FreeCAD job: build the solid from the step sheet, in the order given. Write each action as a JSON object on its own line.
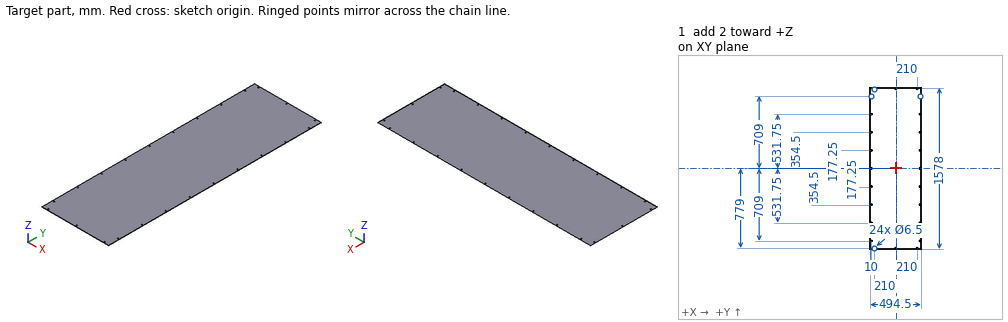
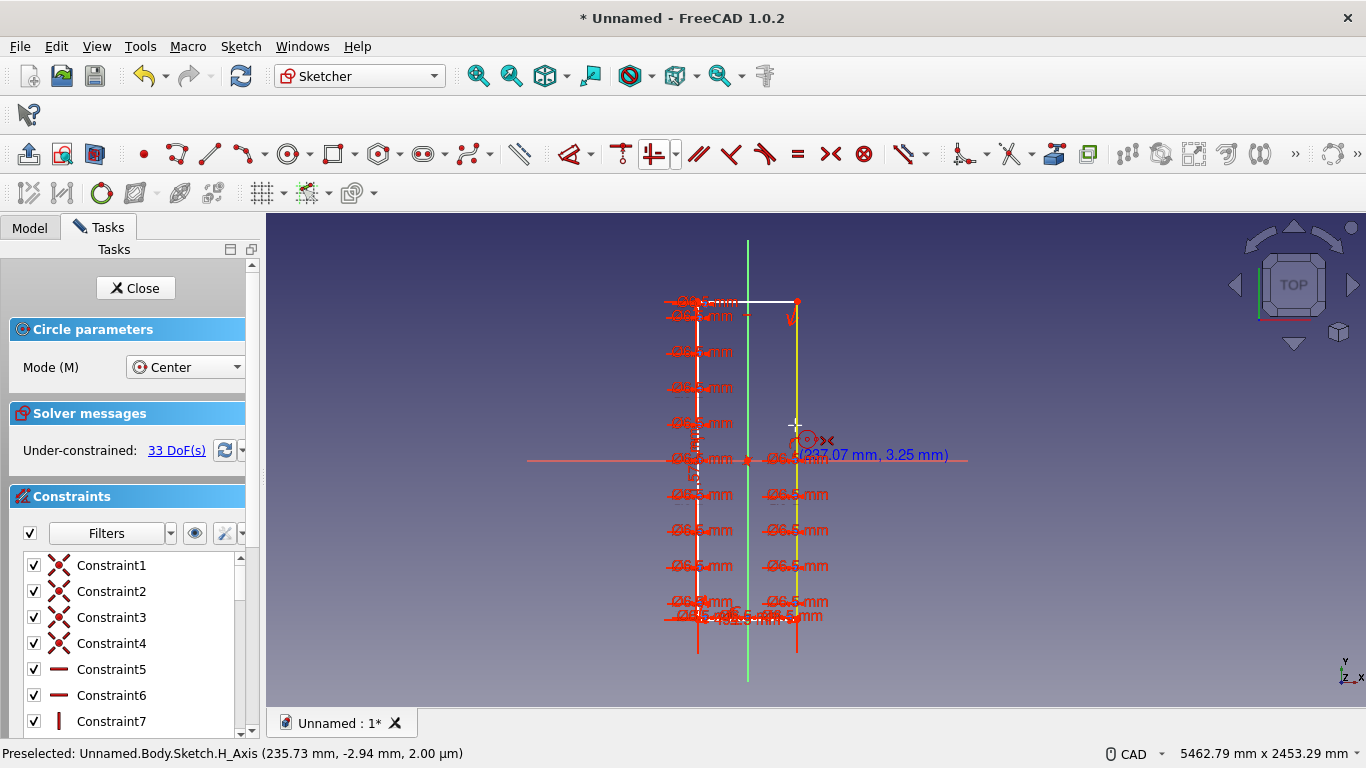
{"action": "scroll", "coordinate": [795, 425], "scroll_direction": "up", "scroll_amount": 11}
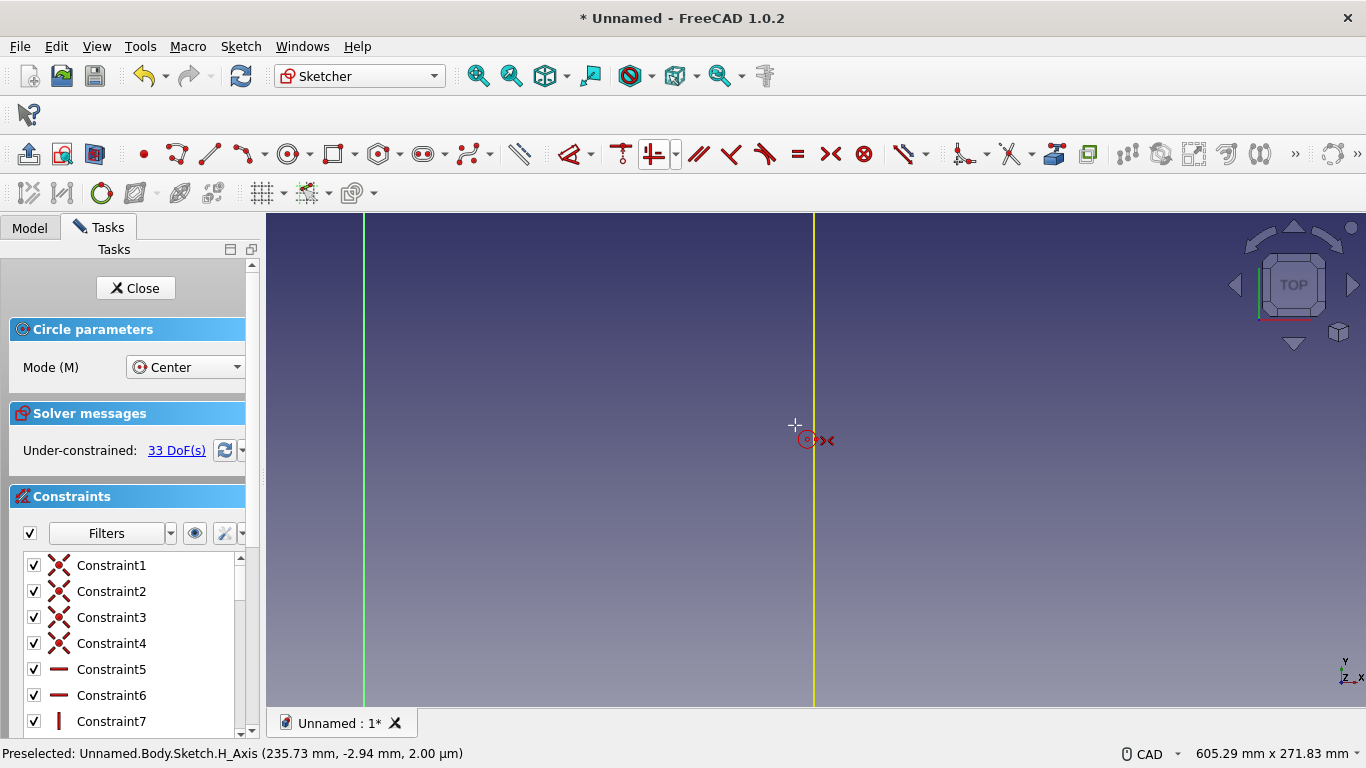
{"action": "left_click", "coordinate": [795, 423]}
{"action": "mouse_move", "coordinate": [791, 419]}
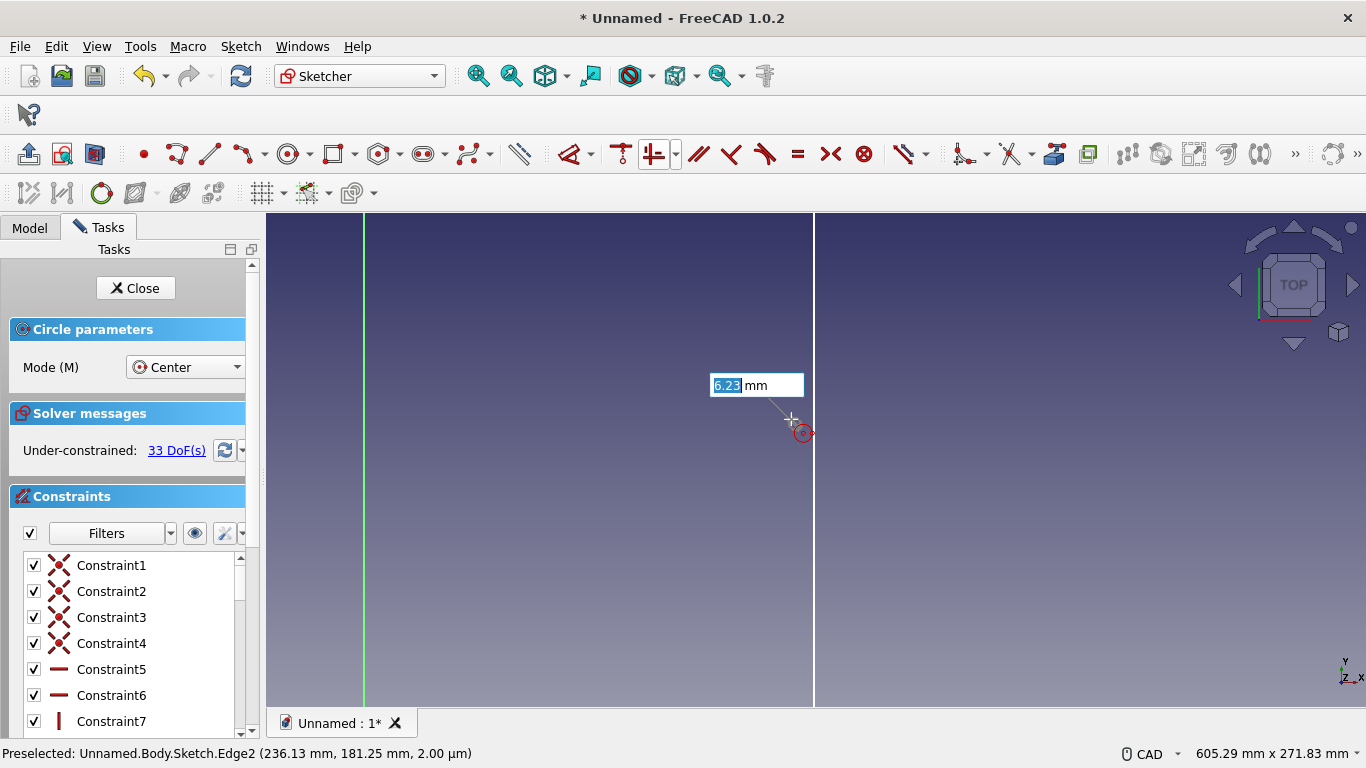
{"action": "type", "text": "6.5"}
{"action": "key", "text": "Return"}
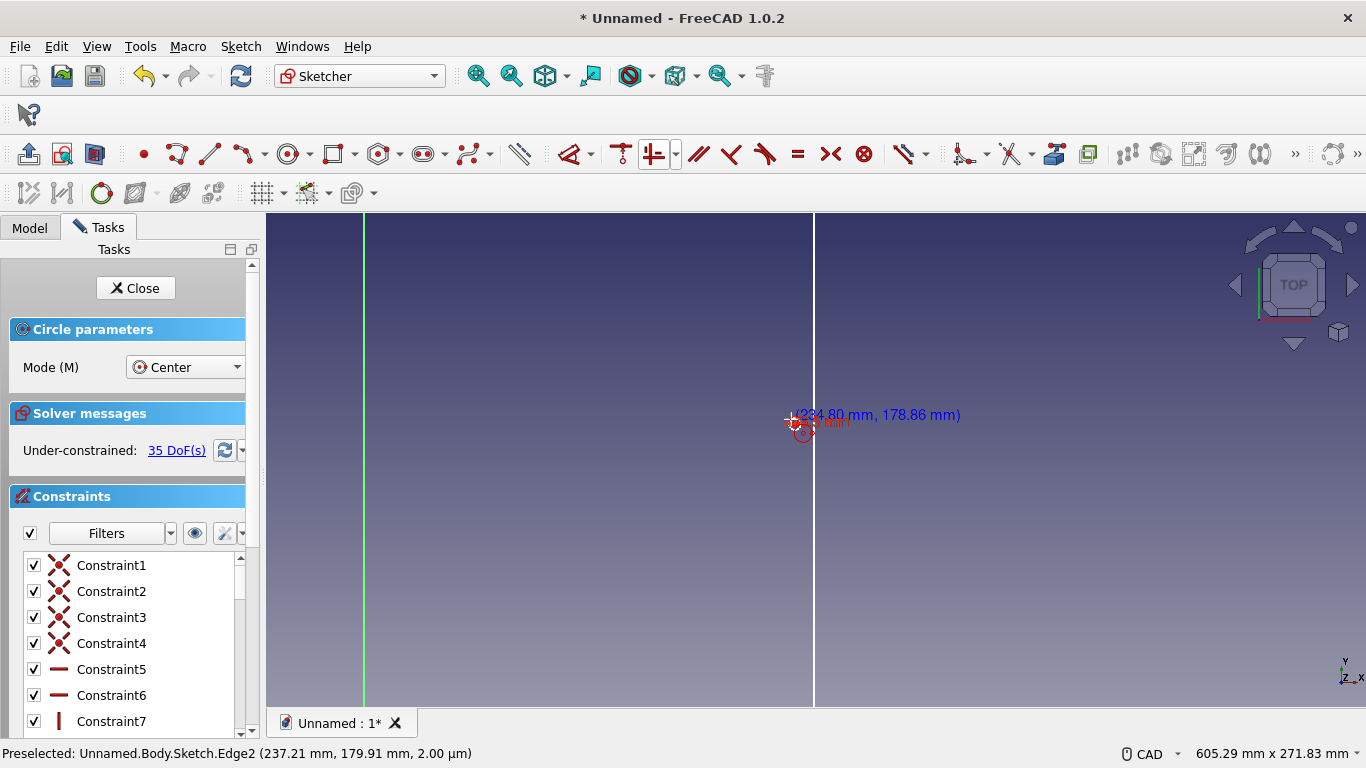
{"action": "scroll", "coordinate": [795, 424], "scroll_direction": "down", "scroll_amount": 11}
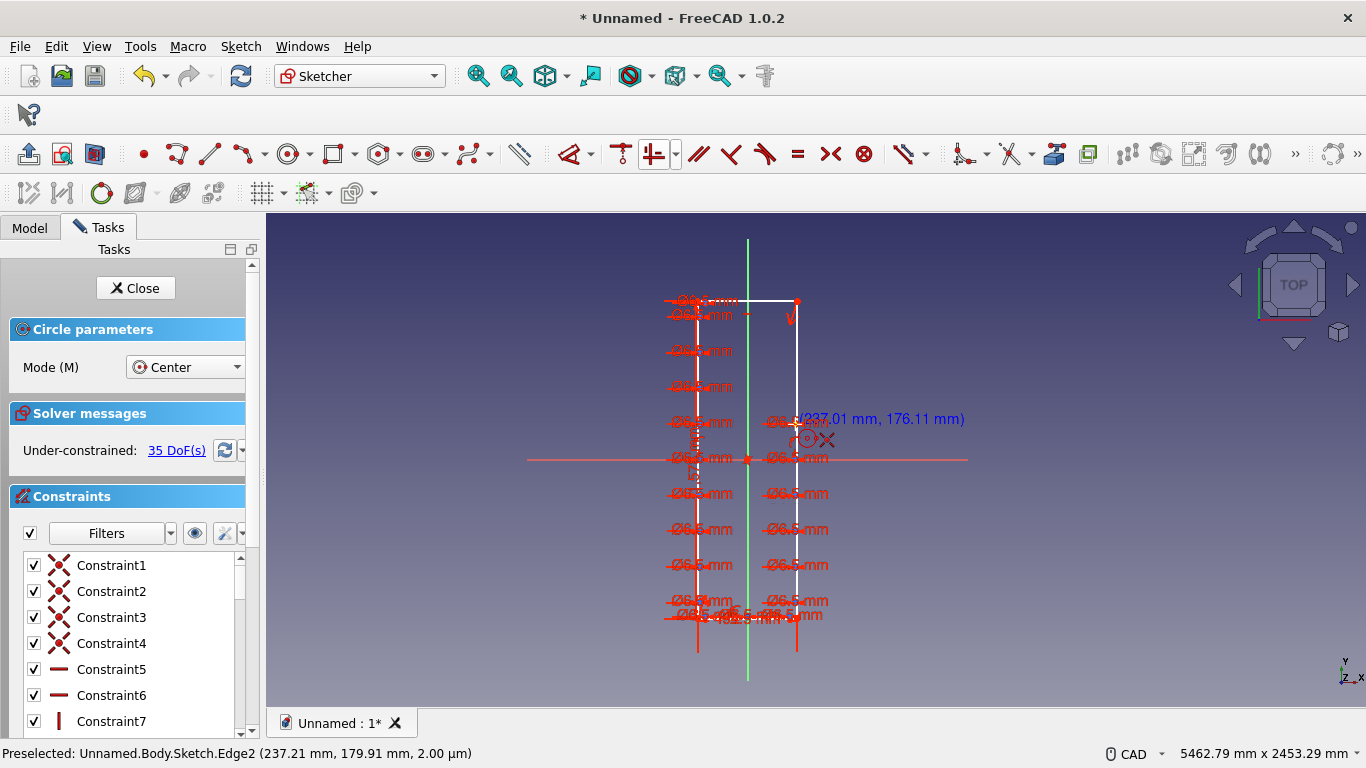
{"action": "scroll", "coordinate": [795, 389], "scroll_direction": "up", "scroll_amount": 18}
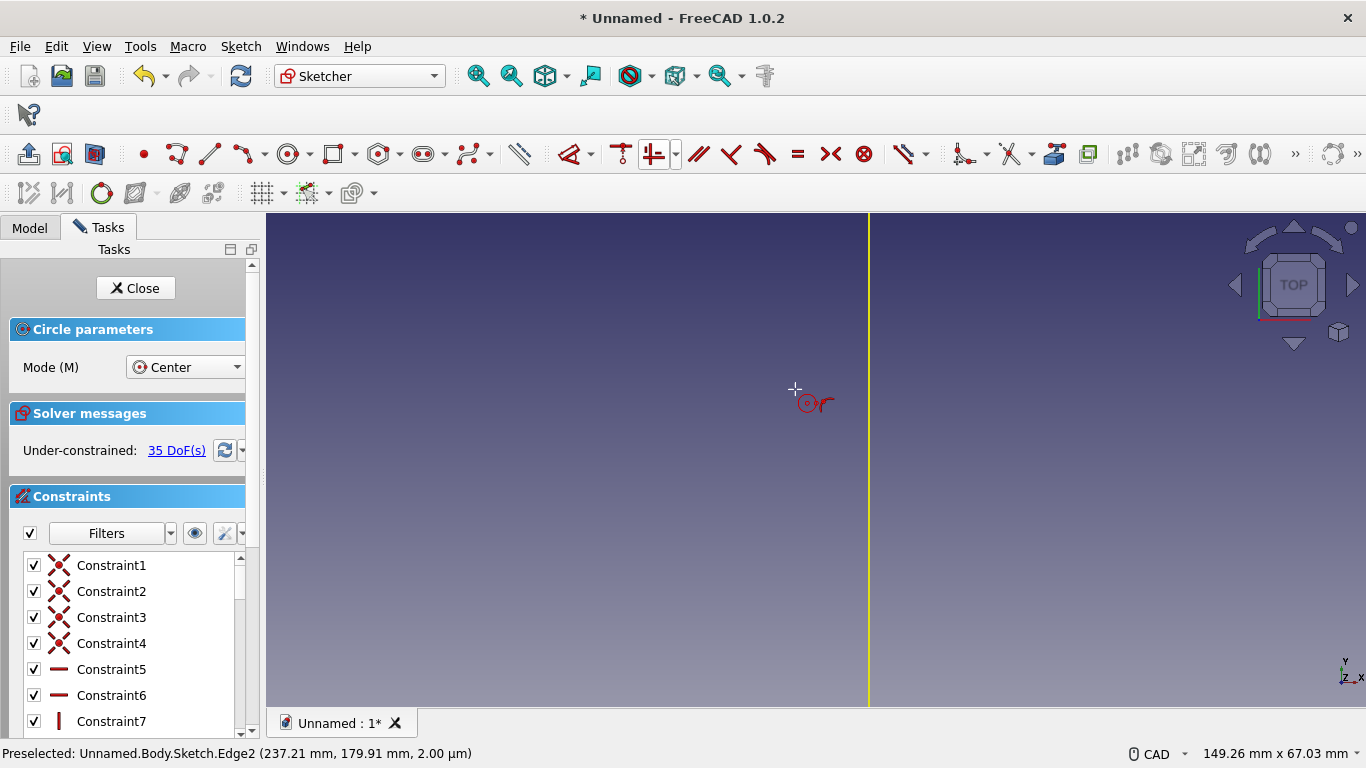
{"action": "scroll", "coordinate": [795, 389], "scroll_direction": "down", "scroll_amount": 18}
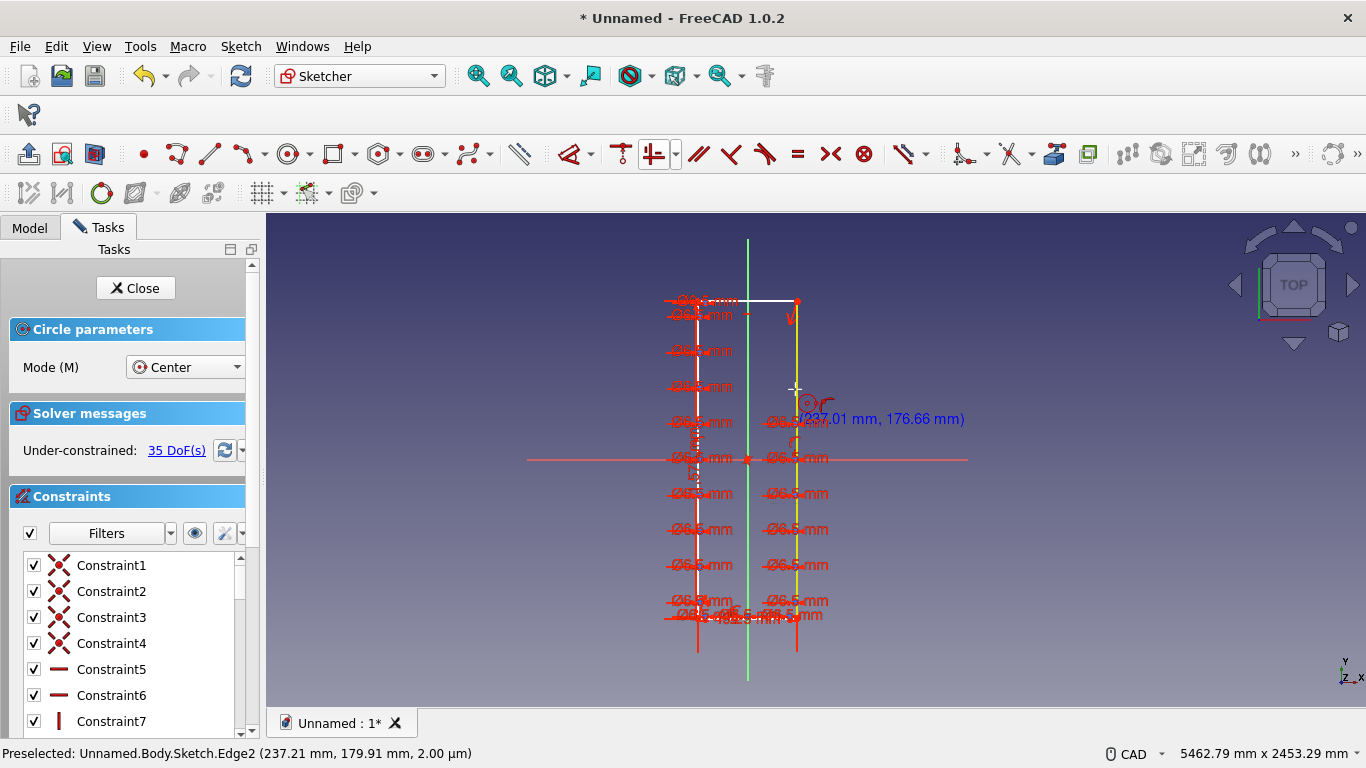
{"action": "scroll", "coordinate": [795, 389], "scroll_direction": "up", "scroll_amount": 11}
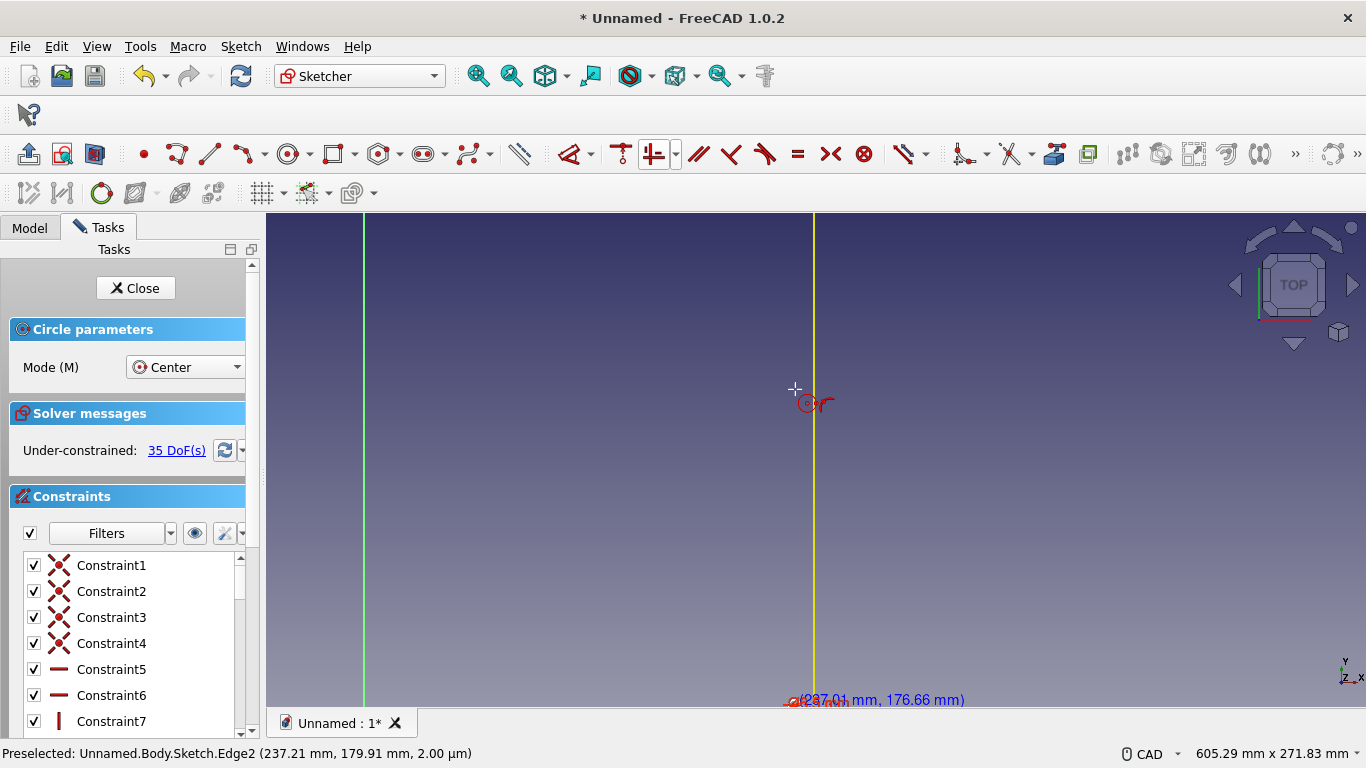
{"action": "left_click", "coordinate": [795, 382]}
{"action": "mouse_move", "coordinate": [791, 378]}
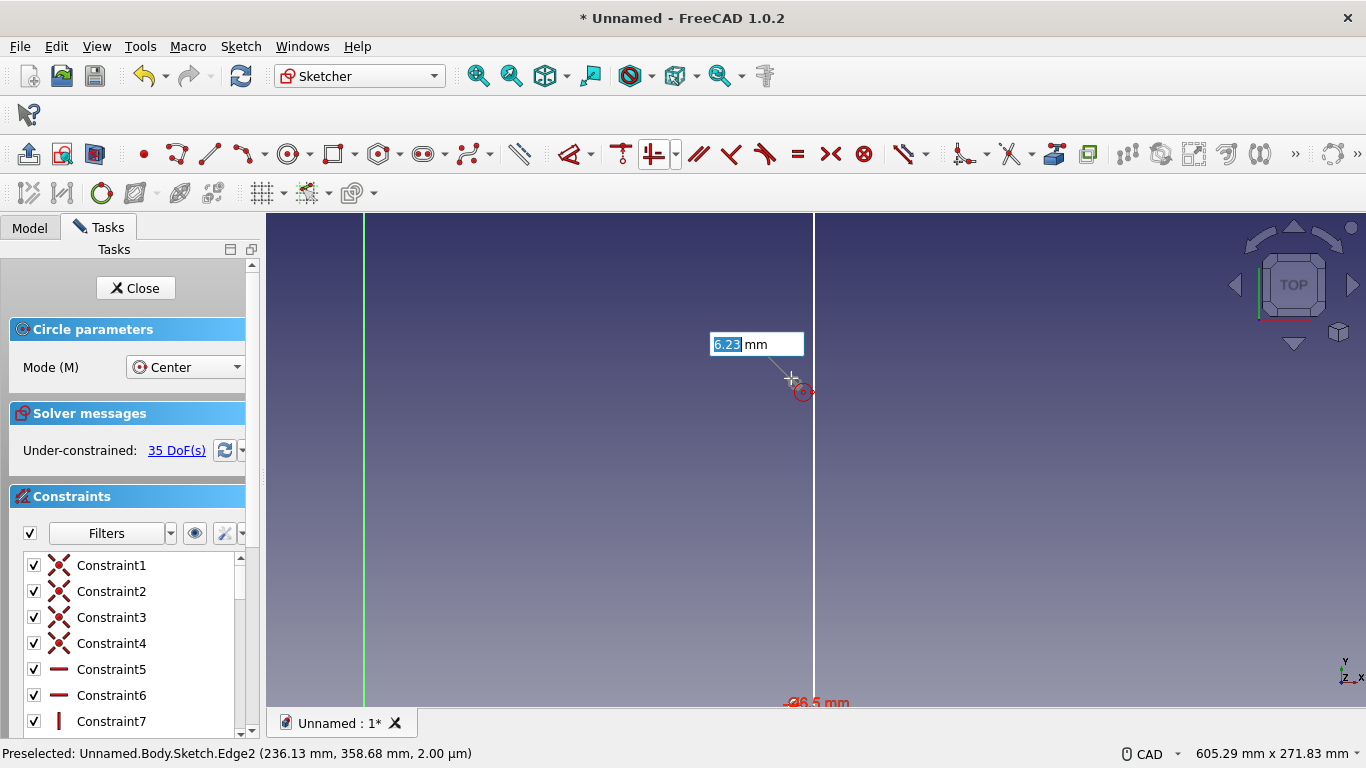
{"action": "type", "text": "6.5"}
{"action": "key", "text": "Return"}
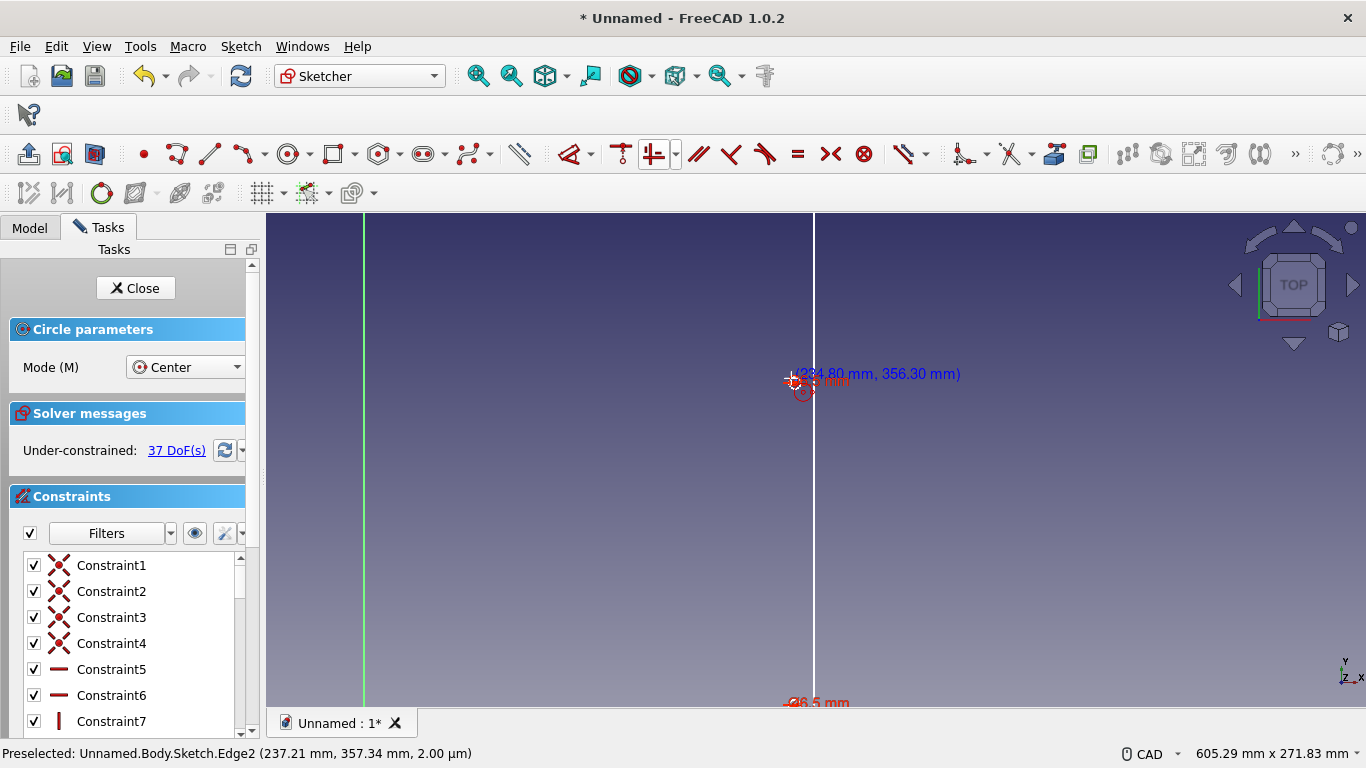
{"action": "scroll", "coordinate": [795, 389], "scroll_direction": "down", "scroll_amount": 11}